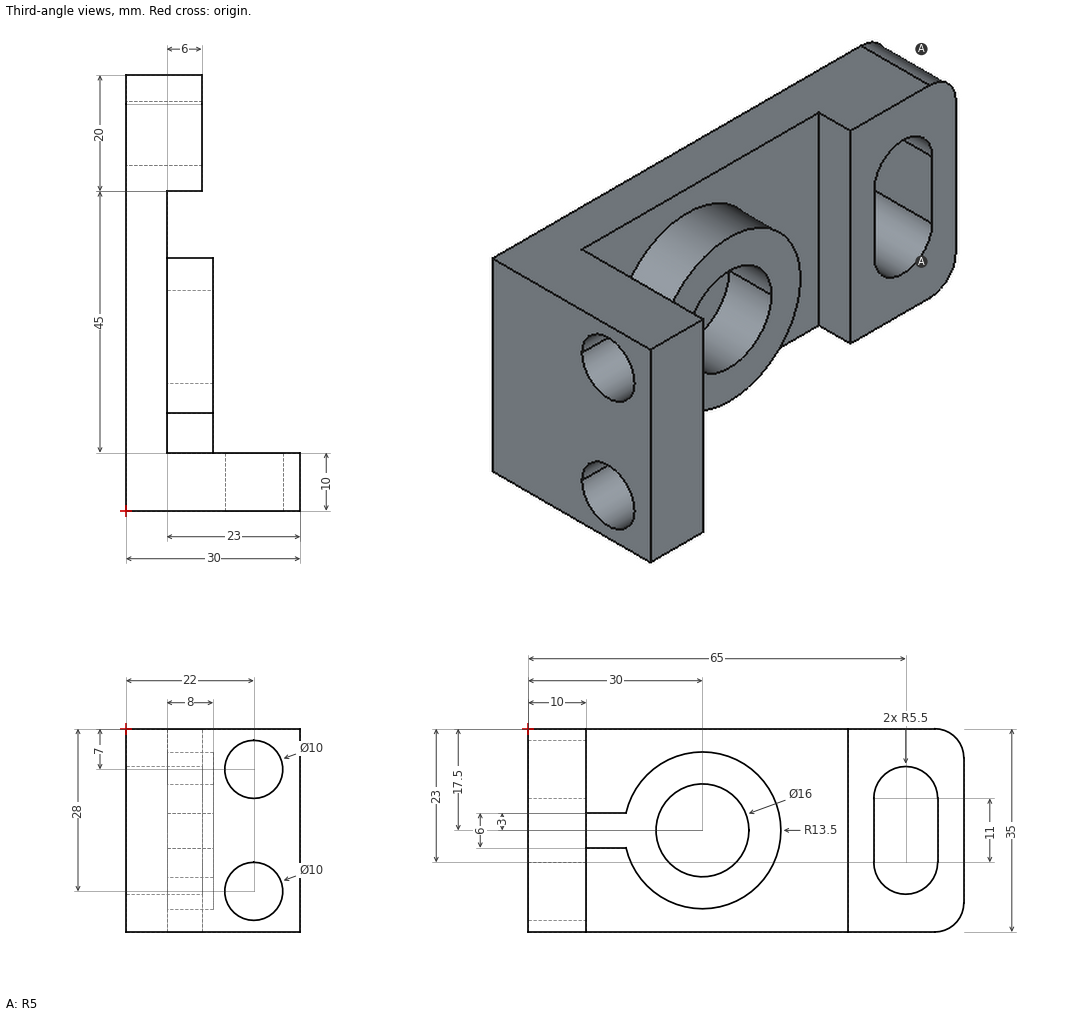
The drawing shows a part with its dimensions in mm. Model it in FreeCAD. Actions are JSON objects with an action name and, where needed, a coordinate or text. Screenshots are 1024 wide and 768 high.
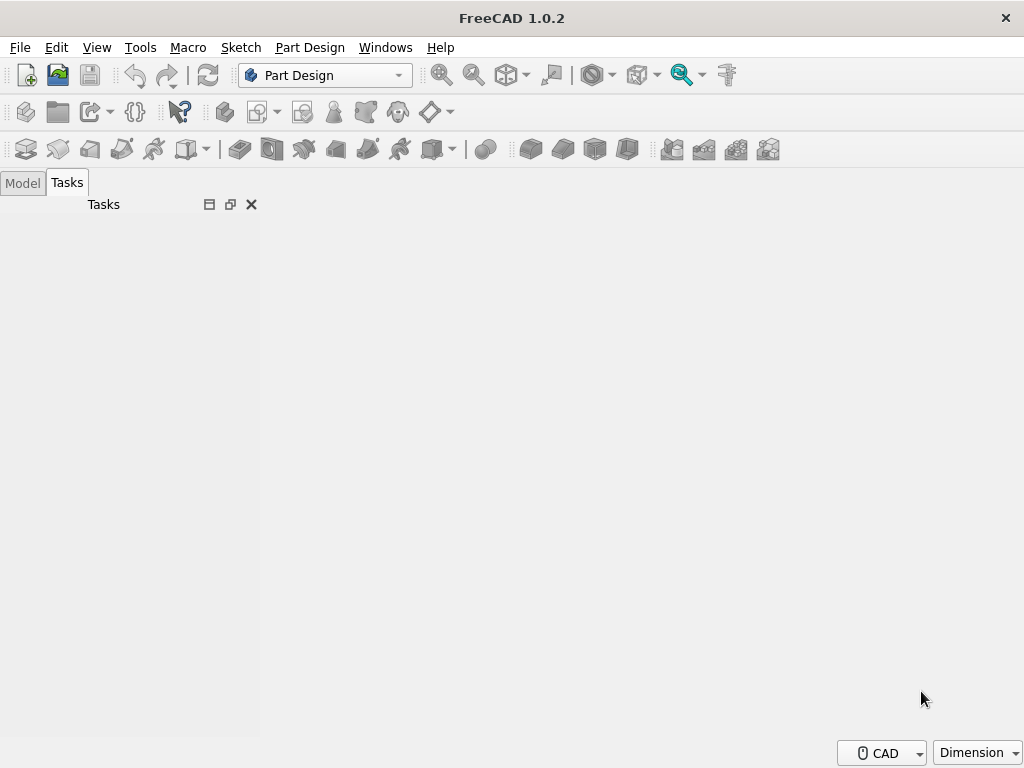
{"action": "left_click", "coordinate": [532, 112]}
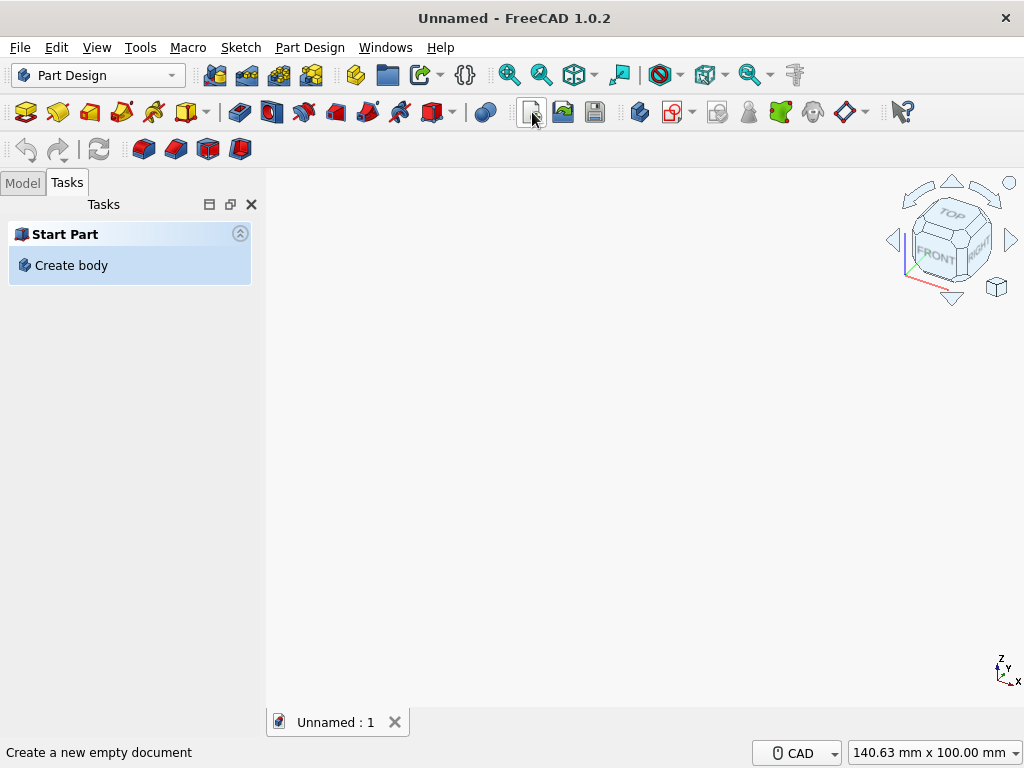
{"action": "left_click", "coordinate": [672, 112]}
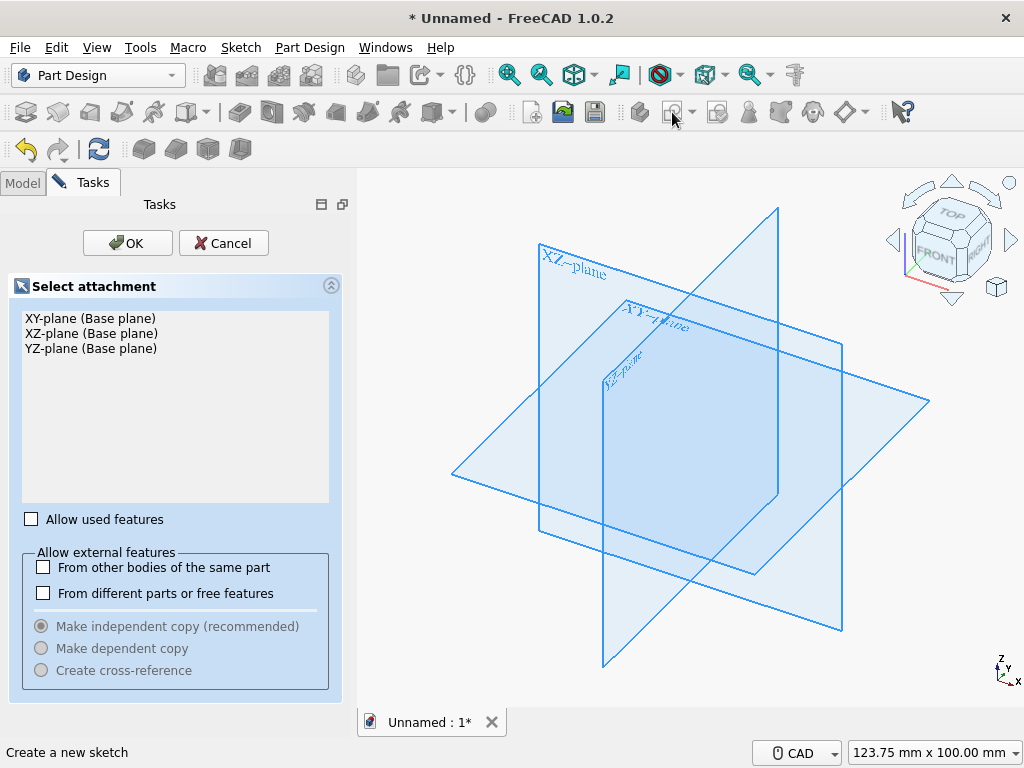
{"action": "left_click", "coordinate": [82, 318]}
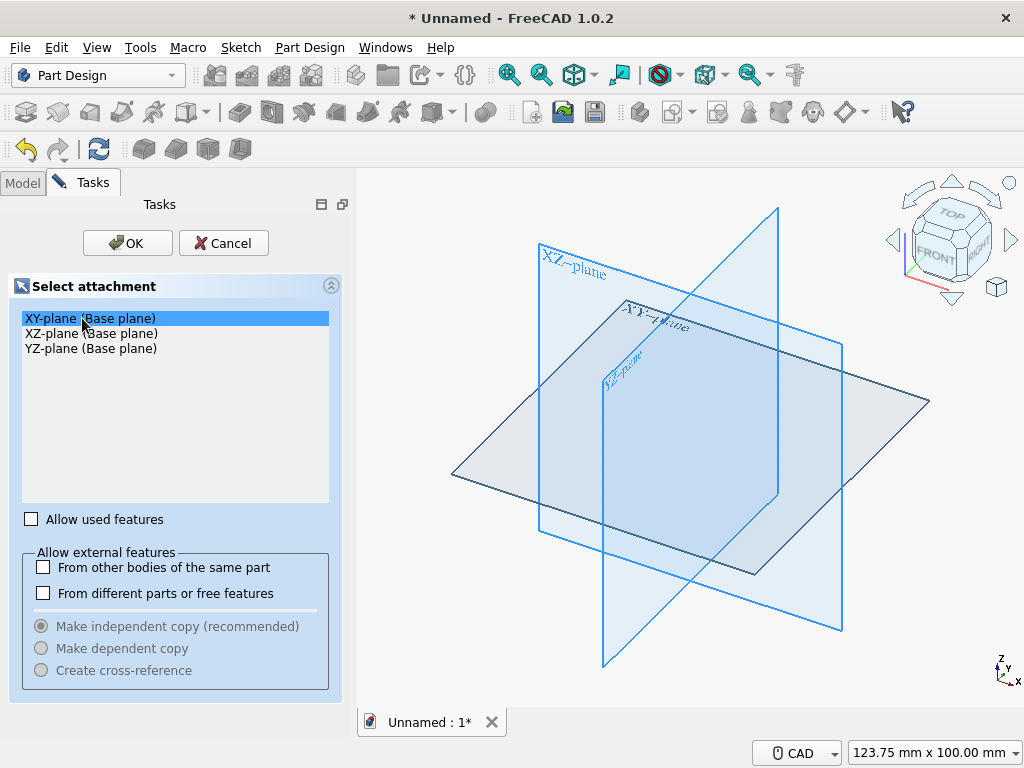
{"action": "left_click", "coordinate": [128, 243]}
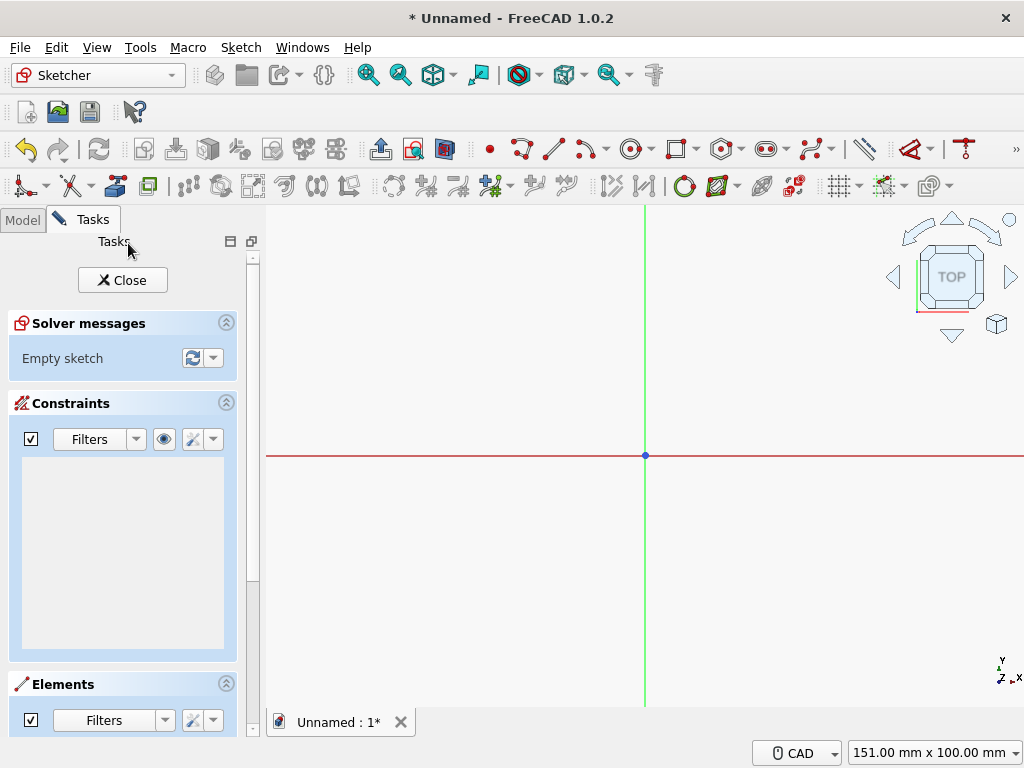
{"action": "scroll", "coordinate": [294, 679], "scroll_direction": "down", "scroll_amount": 2}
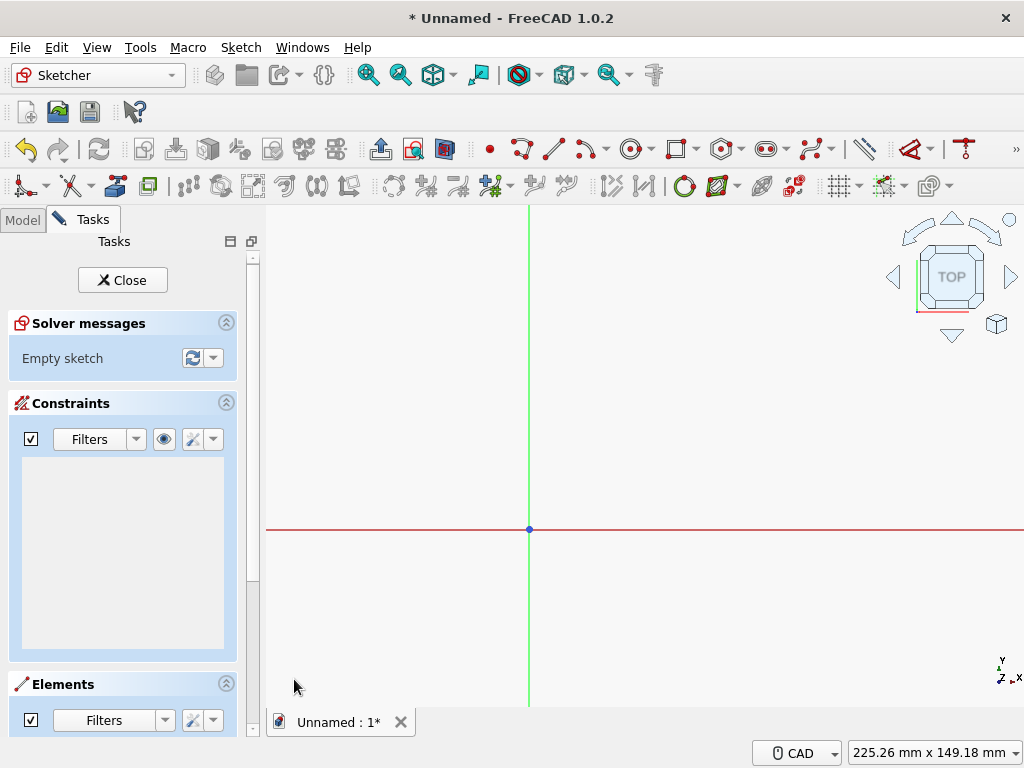
{"action": "key", "text": "g m"}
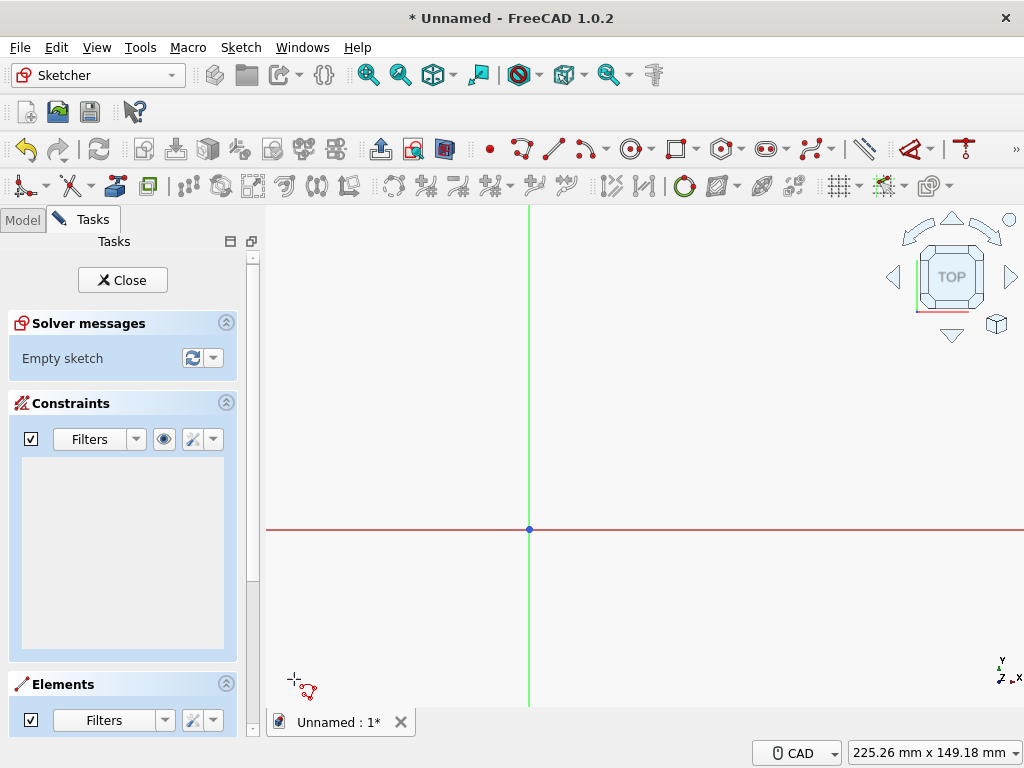
{"action": "left_click", "coordinate": [529, 530]}
{"action": "left_click", "coordinate": [630, 521]}
{"action": "left_click", "coordinate": [630, 496]}
{"action": "left_click", "coordinate": [553, 496]}
{"action": "left_click", "coordinate": [553, 345]}
{"action": "left_click", "coordinate": [573, 345]}
{"action": "left_click", "coordinate": [573, 277]}
{"action": "left_click", "coordinate": [538, 277]}
{"action": "left_click", "coordinate": [529, 530]}
{"action": "key", "text": "Escape"}
{"action": "key", "text": "Escape"}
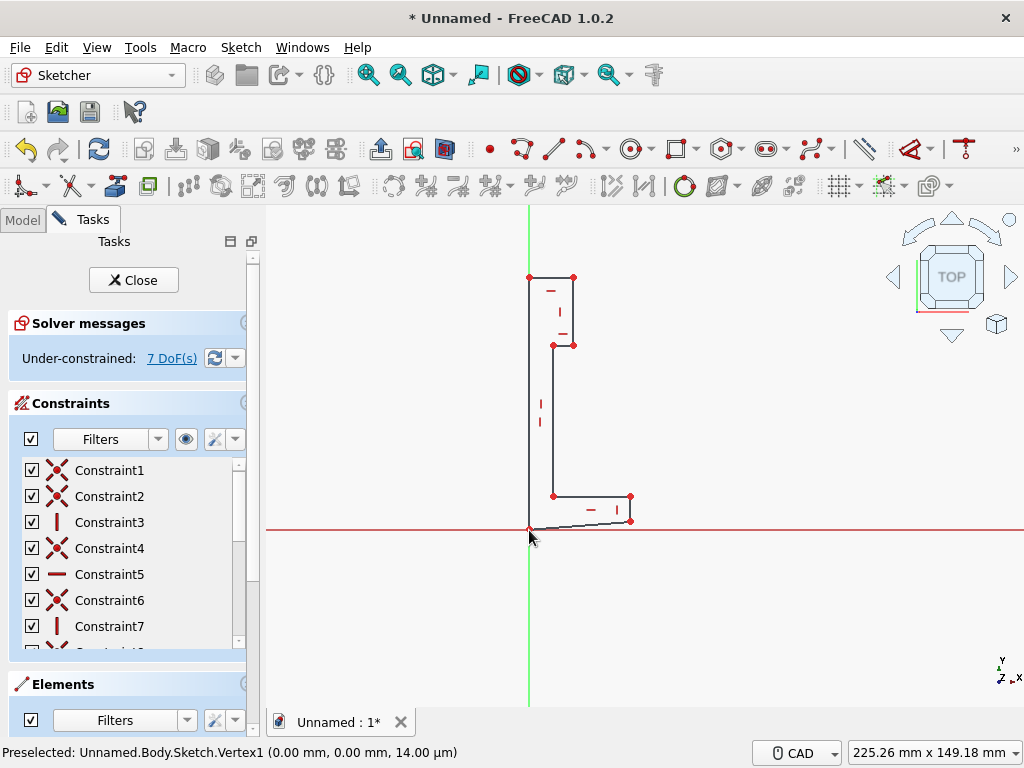
{"action": "left_click", "coordinate": [560, 527]}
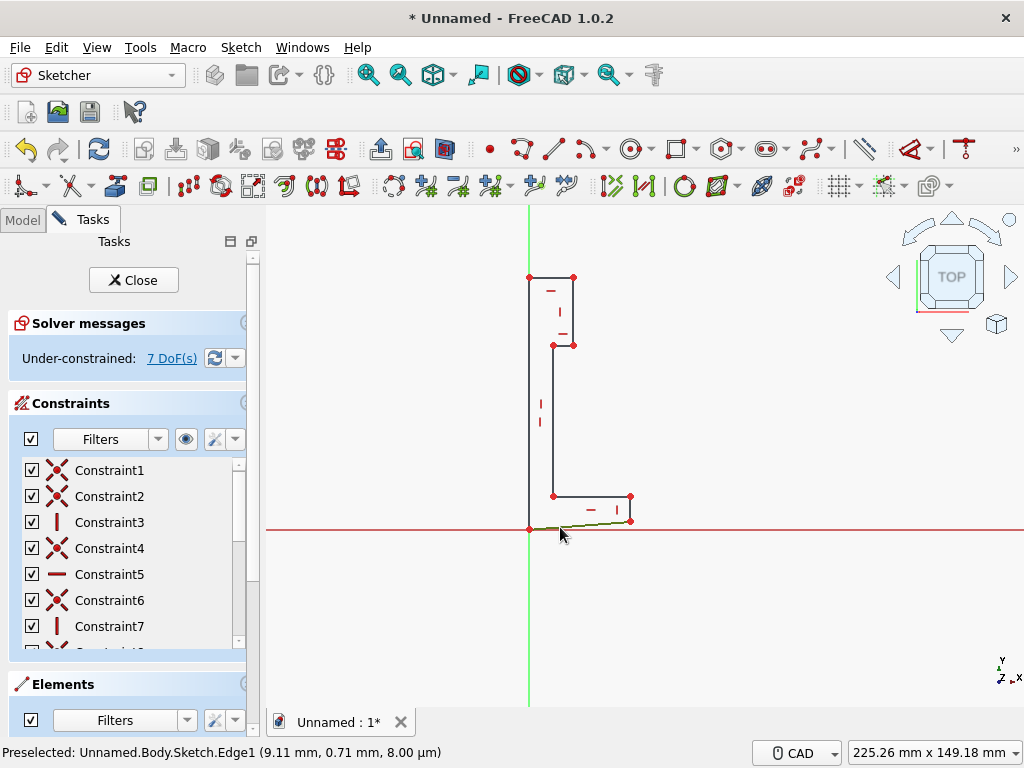
{"action": "key", "text": "h"}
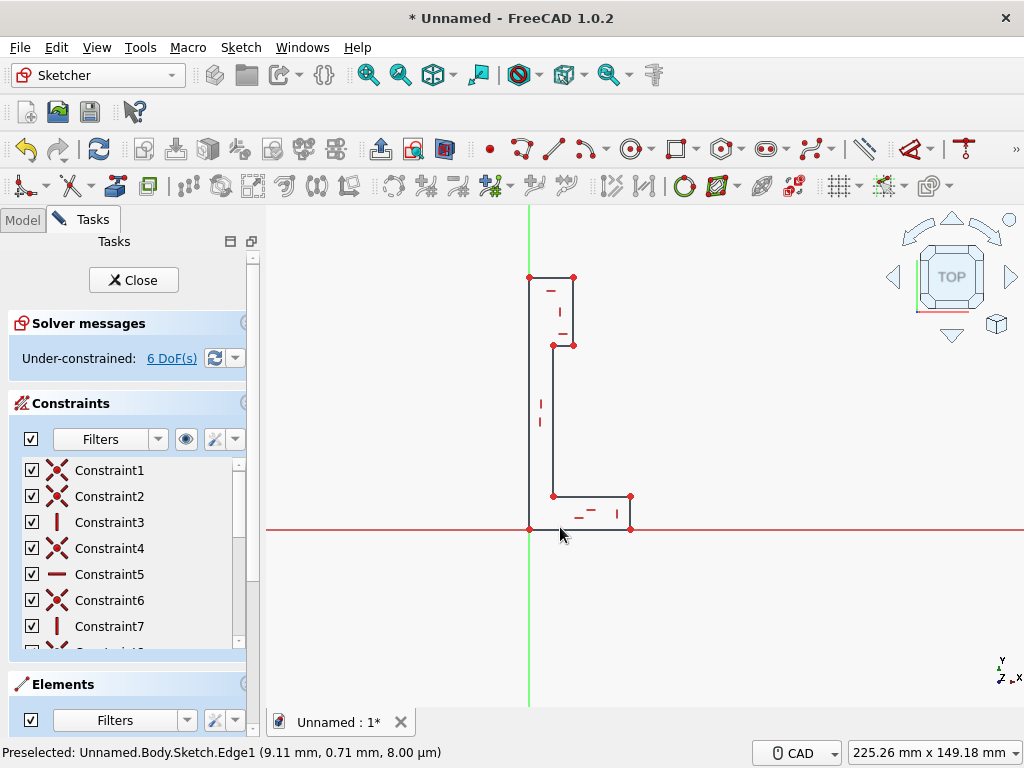
{"action": "left_click", "coordinate": [910, 150]}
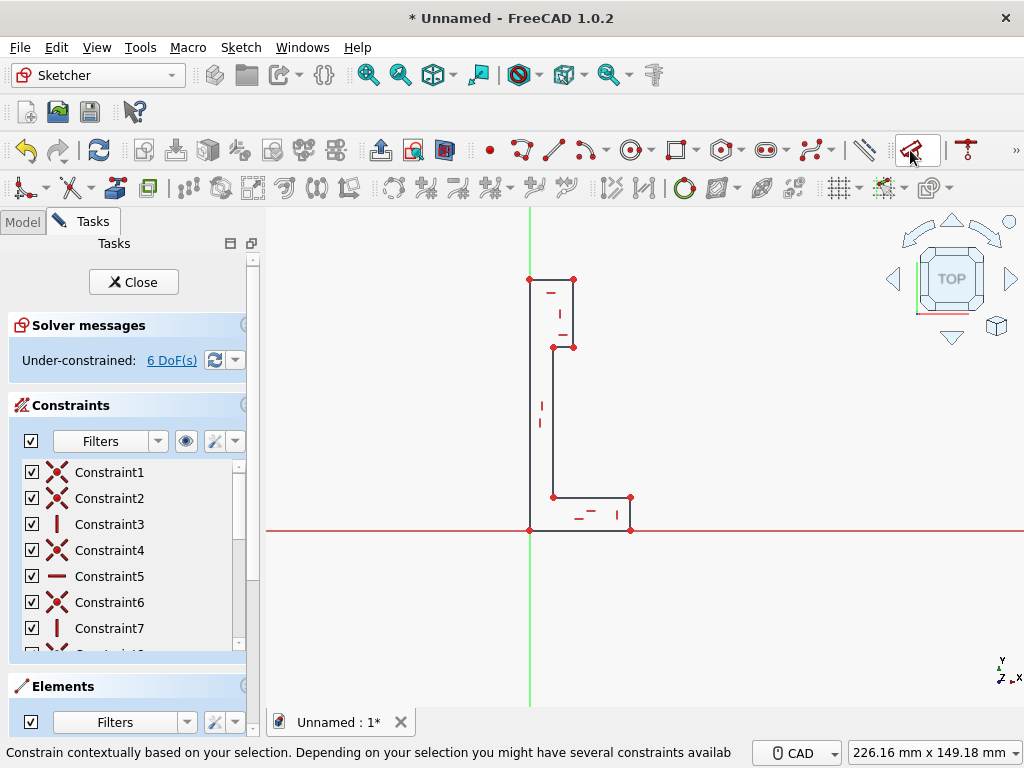
{"action": "scroll", "coordinate": [563, 347], "scroll_direction": "up", "scroll_amount": 4}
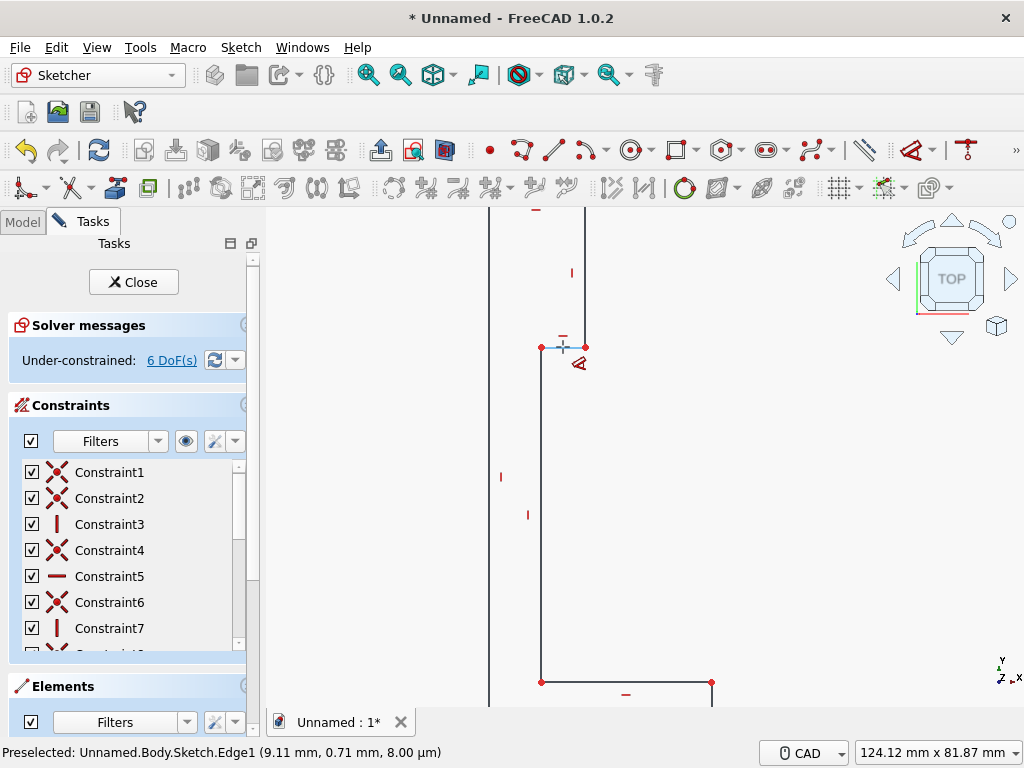
{"action": "left_click", "coordinate": [563, 348]}
{"action": "left_click", "coordinate": [563, 314]}